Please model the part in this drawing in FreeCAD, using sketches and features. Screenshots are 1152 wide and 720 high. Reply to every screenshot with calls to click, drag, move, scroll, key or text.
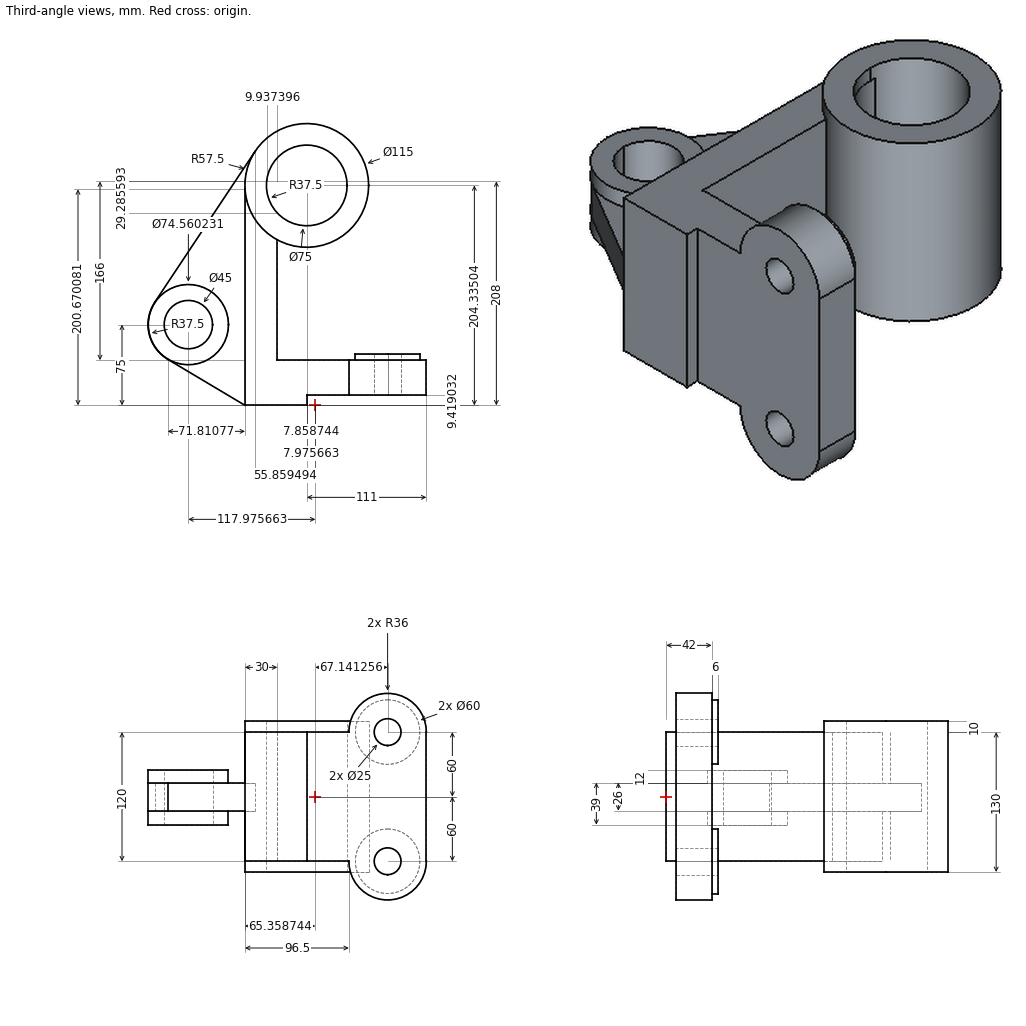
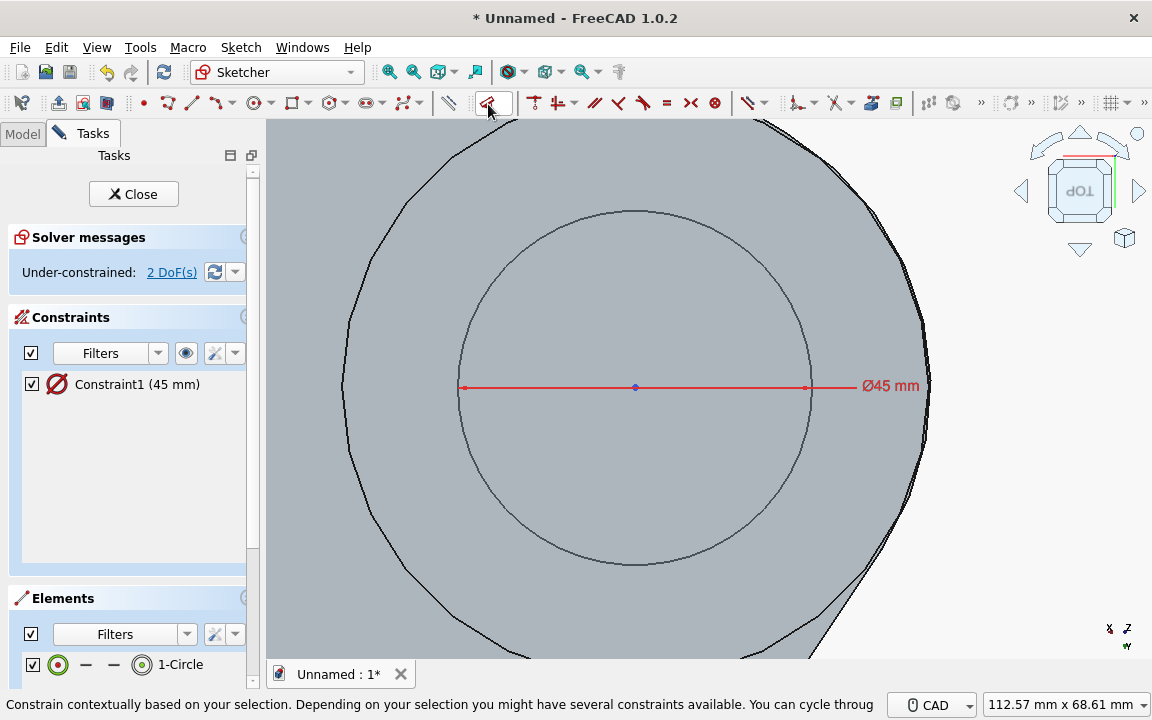
click(635, 388)
click(669, 267)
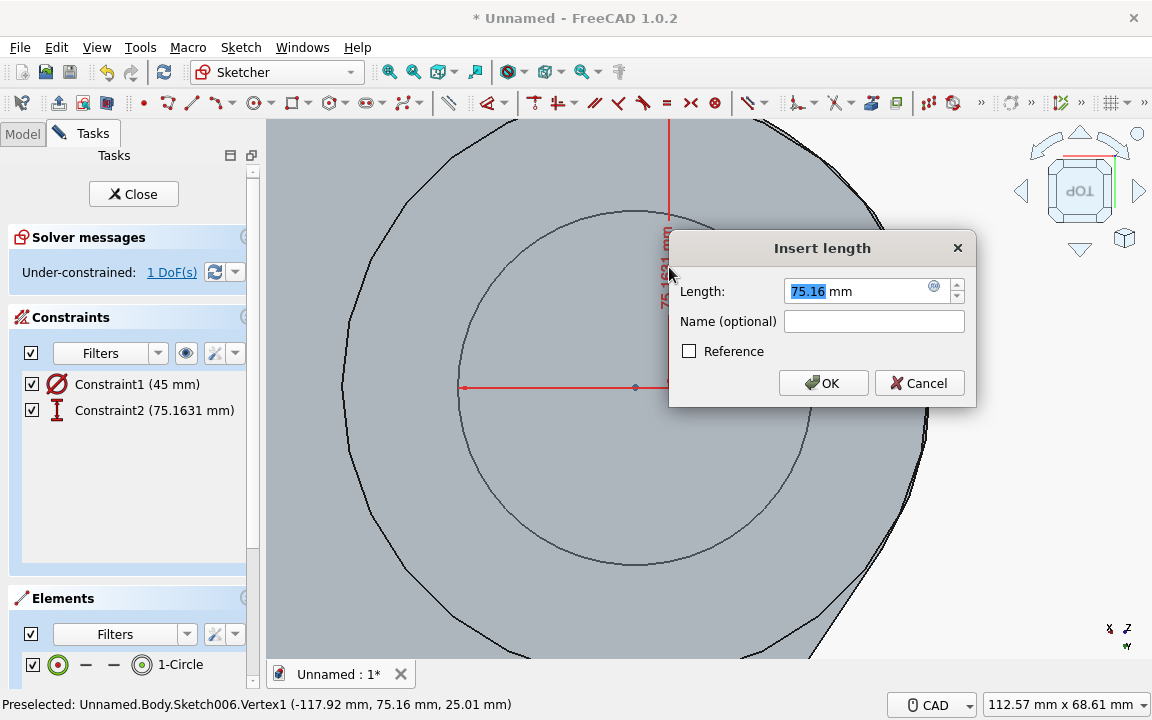
text(75)
key(Return)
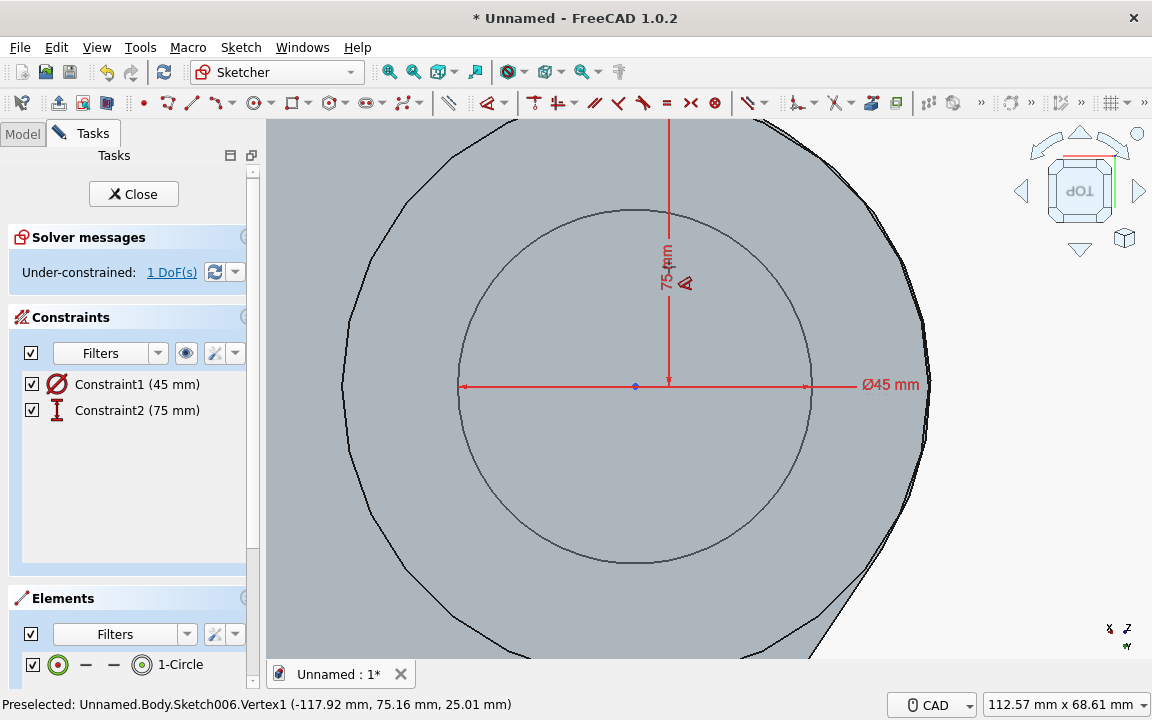
click(635, 387)
click(386, 421)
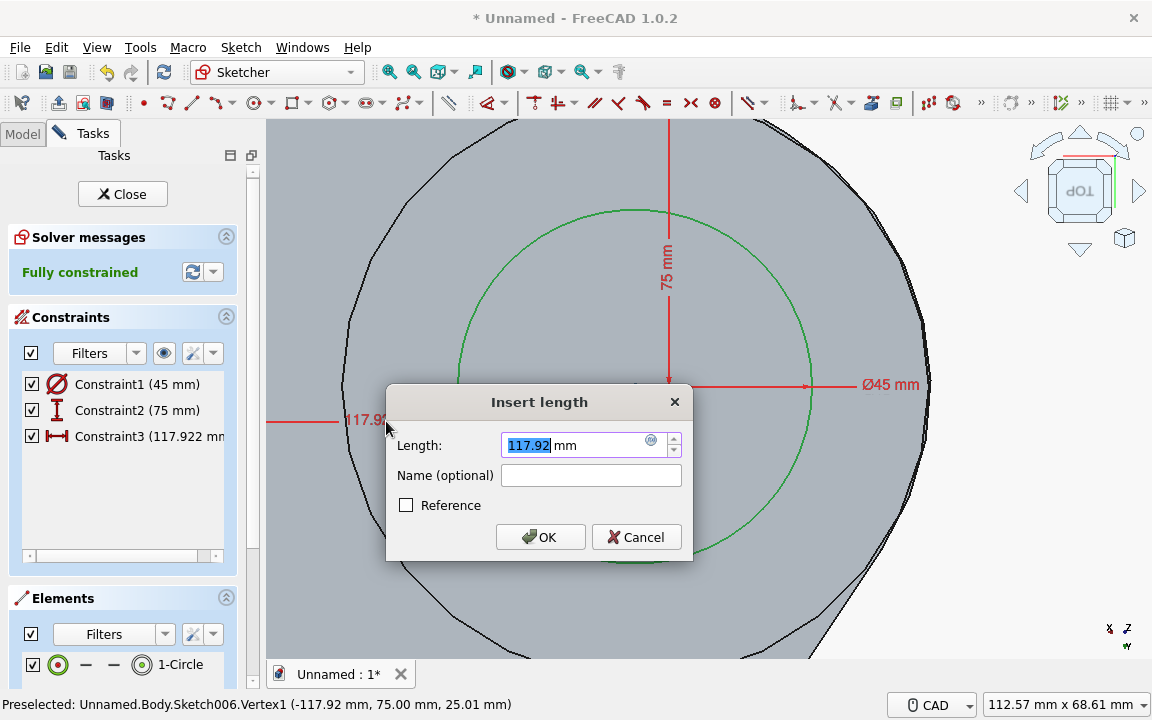
text(117.975663)
key(Return)
key(Escape)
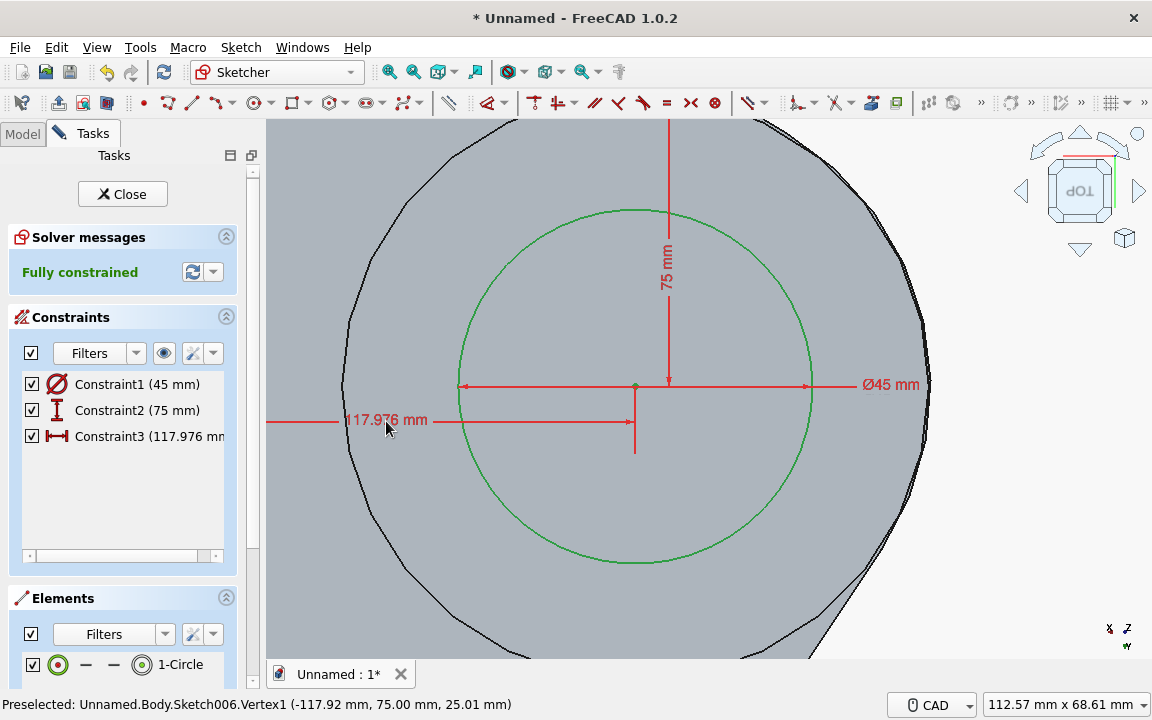
click(123, 194)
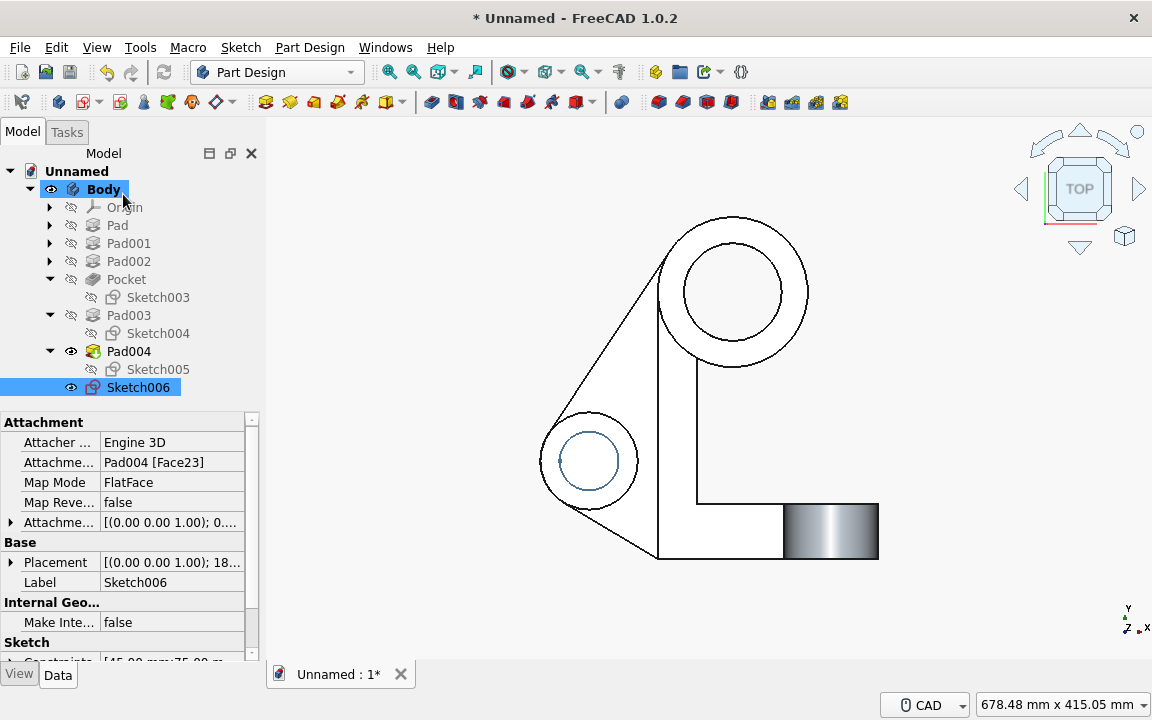
click(432, 102)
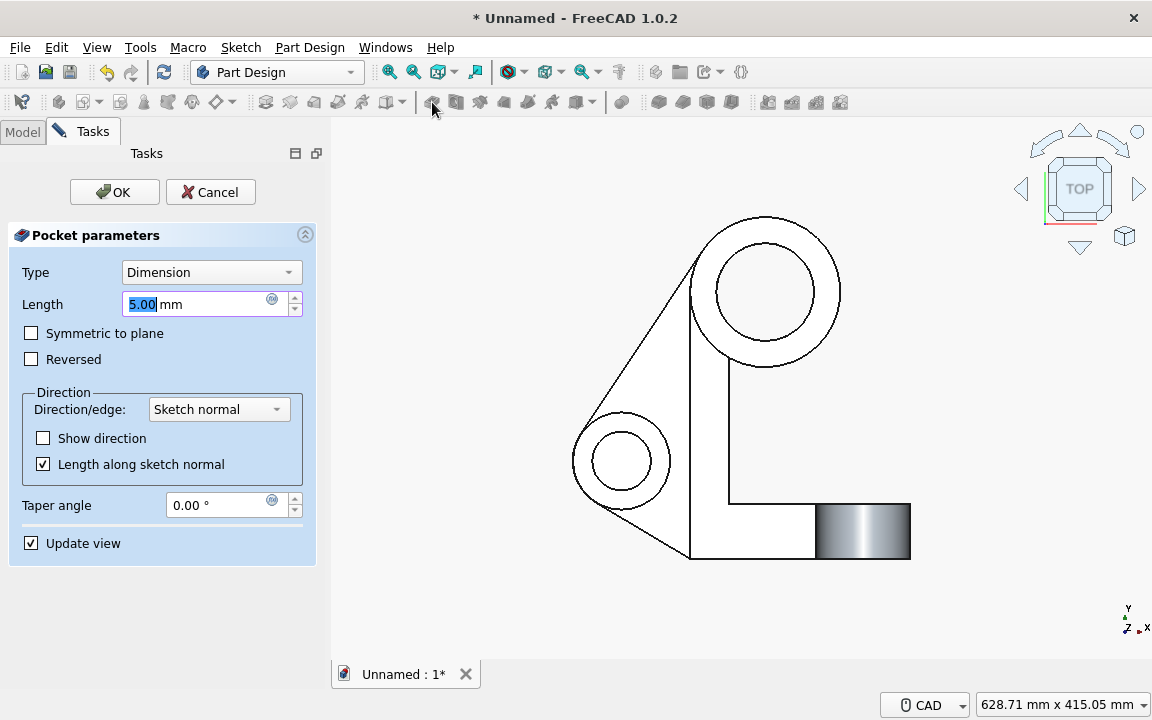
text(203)
key(Tab)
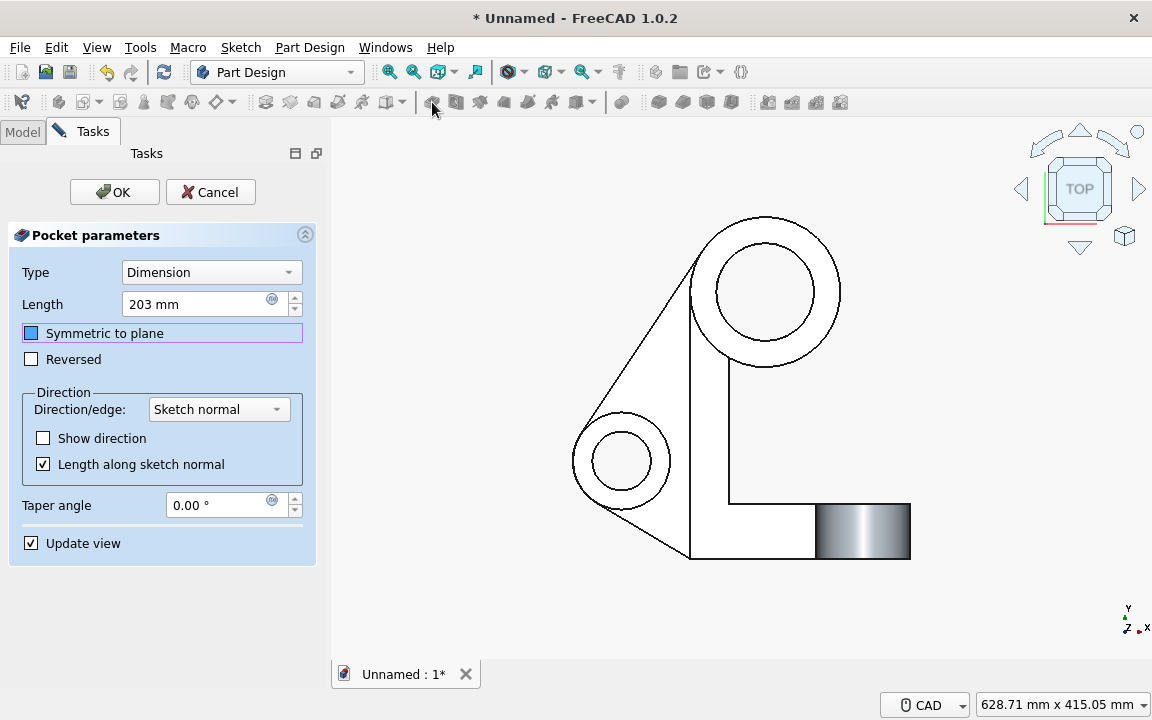
click(115, 192)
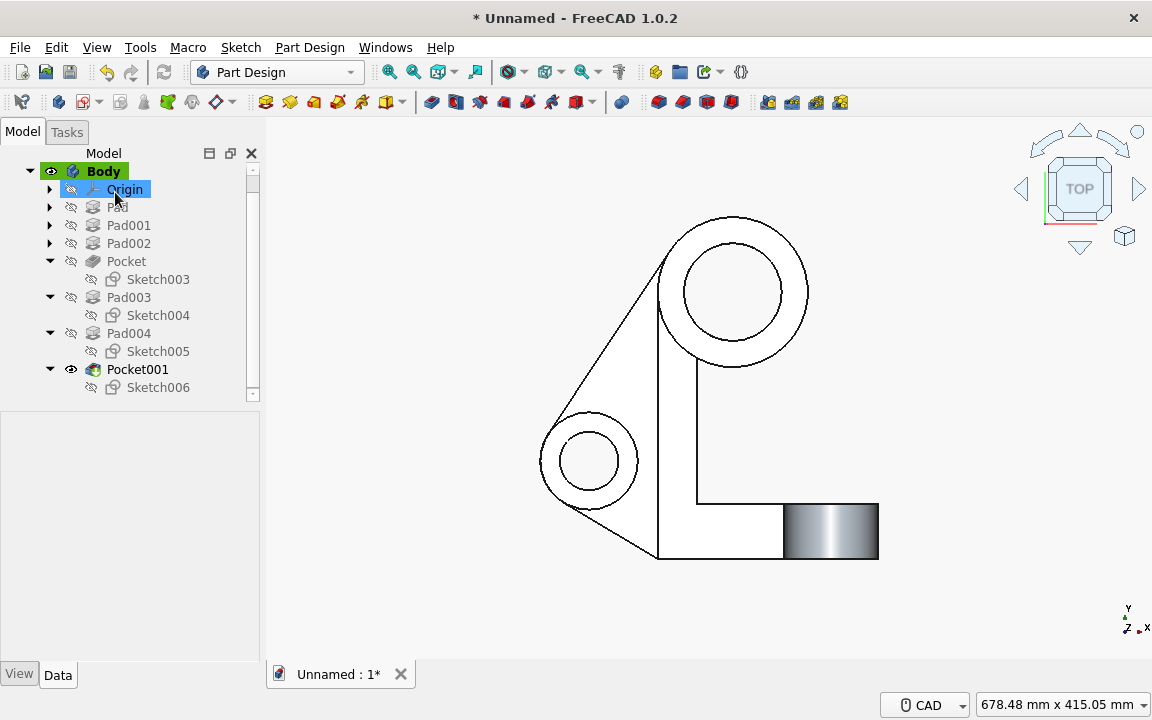
key(4)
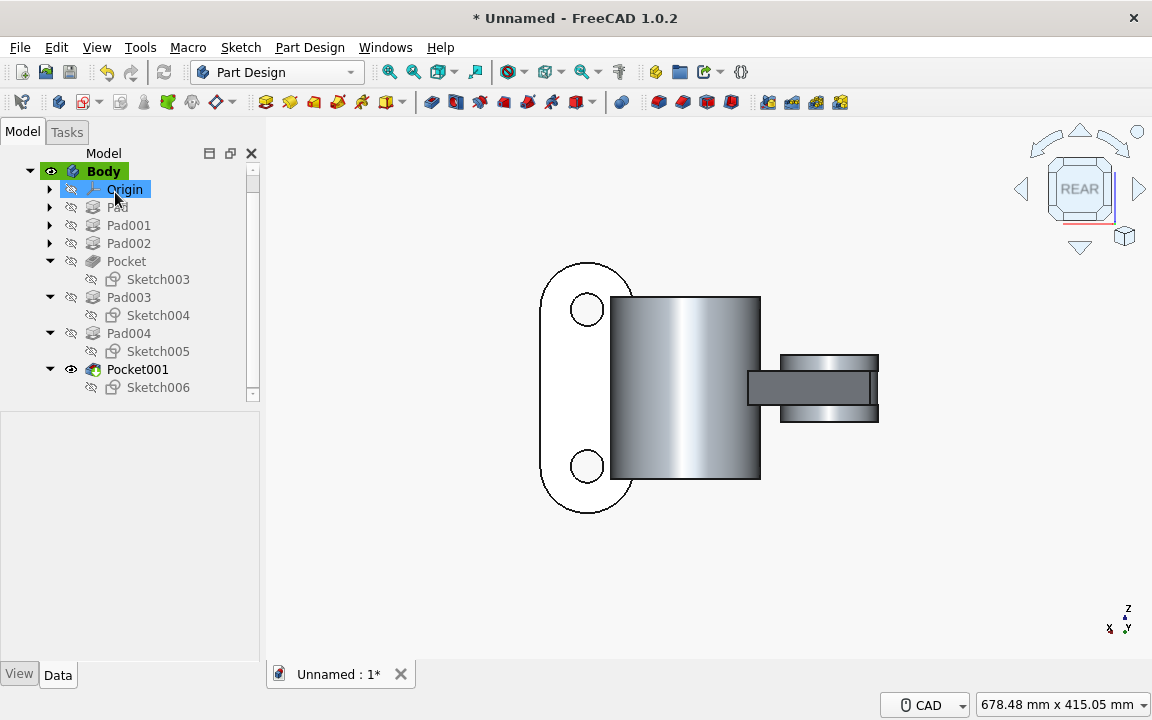
click(605, 387)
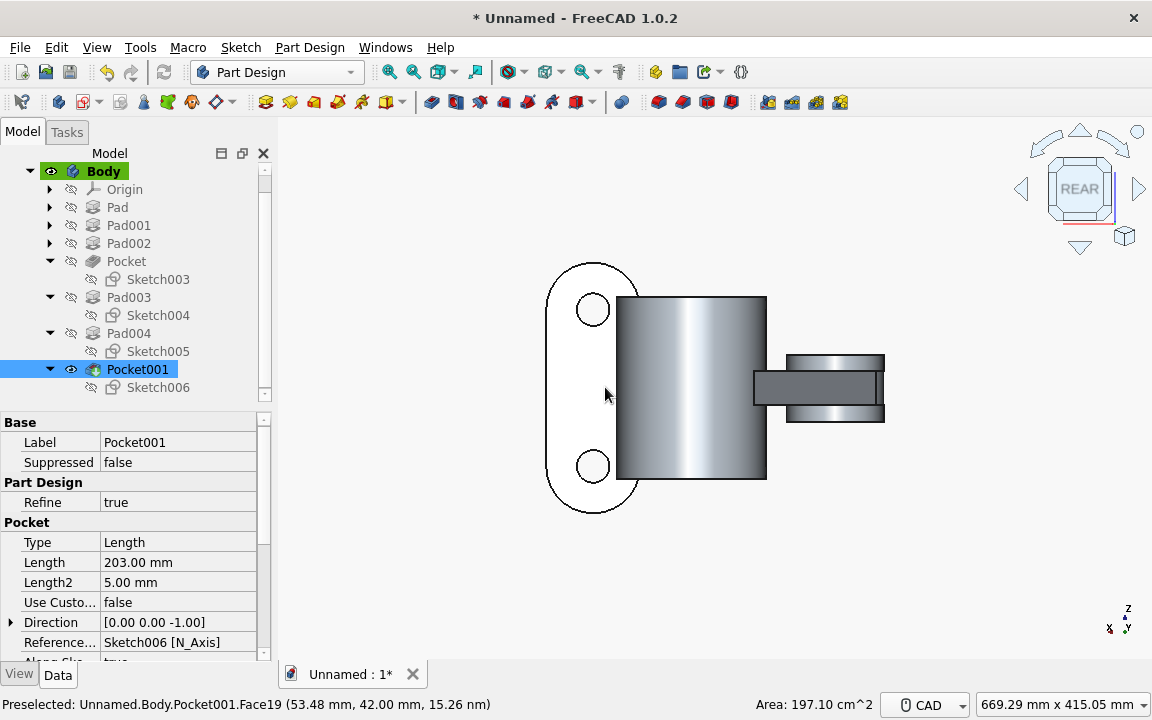
click(84, 102)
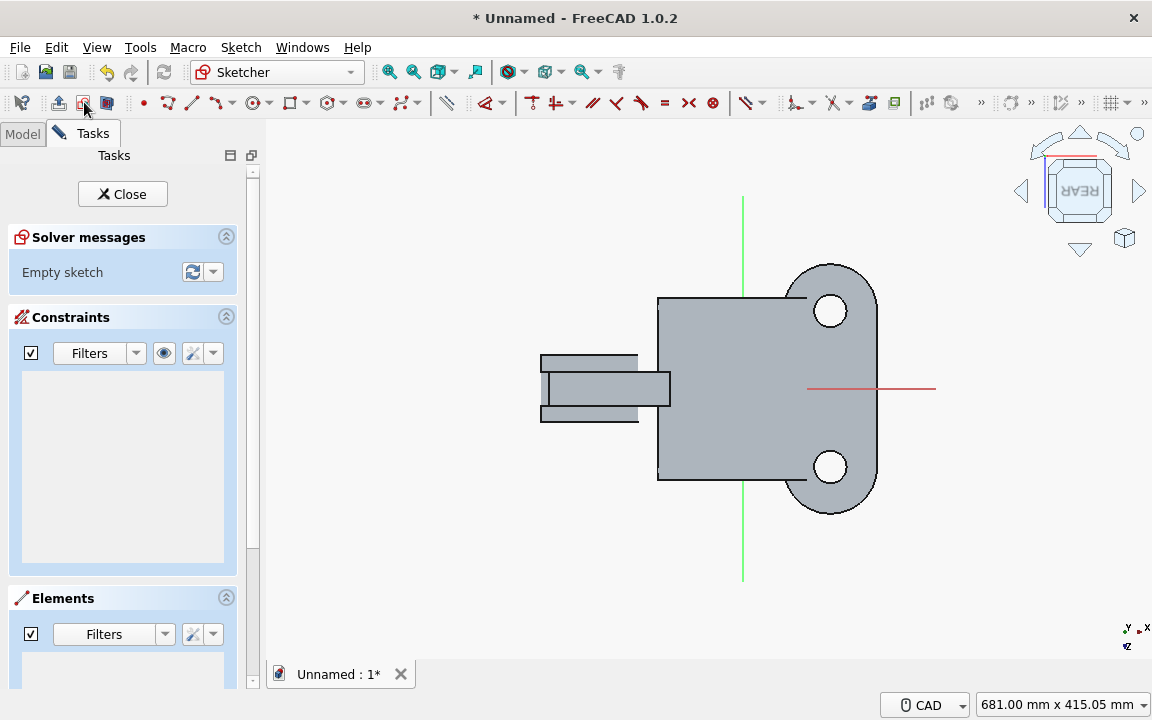
scroll(987, 389, up, 2)